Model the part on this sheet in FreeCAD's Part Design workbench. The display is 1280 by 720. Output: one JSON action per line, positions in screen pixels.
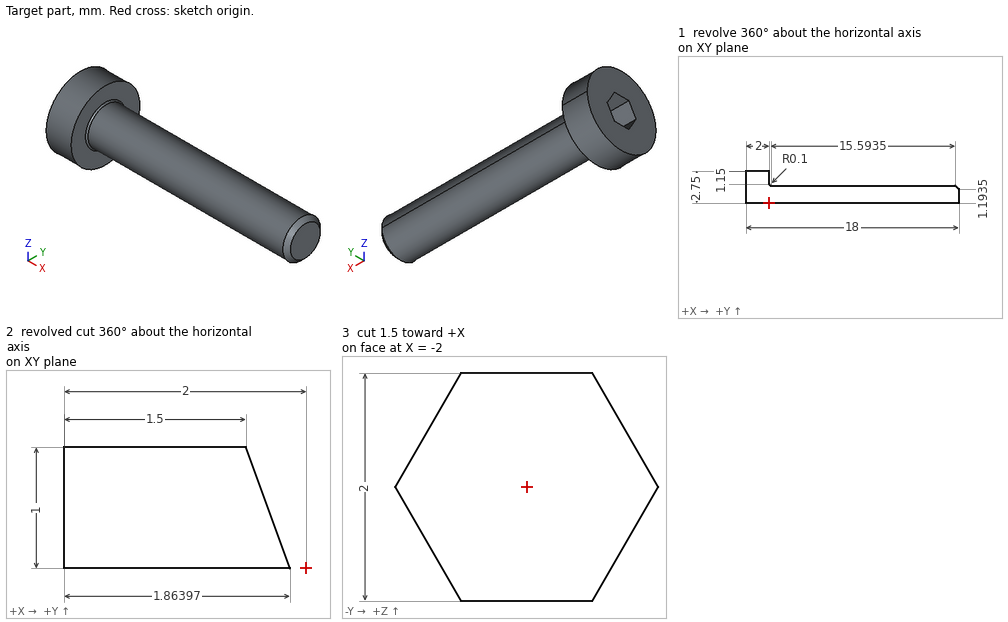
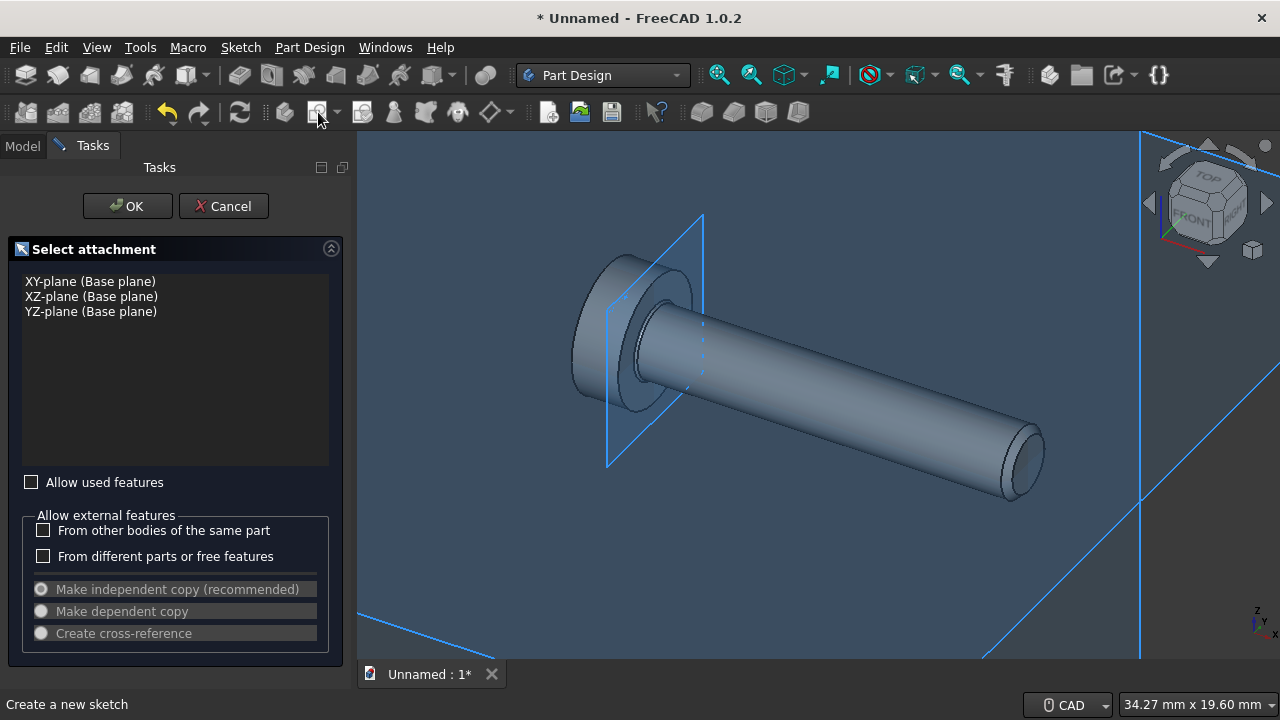
{"action": "left_click", "coordinate": [82, 282]}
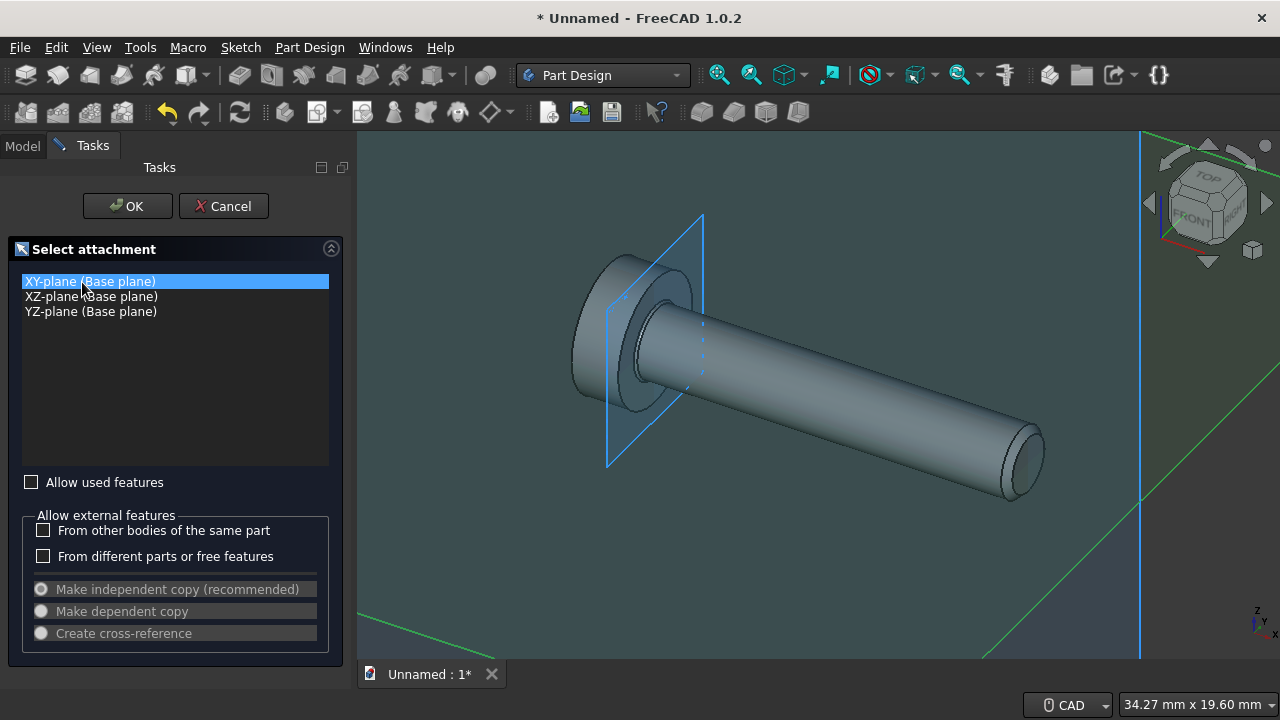
{"action": "left_click", "coordinate": [128, 206]}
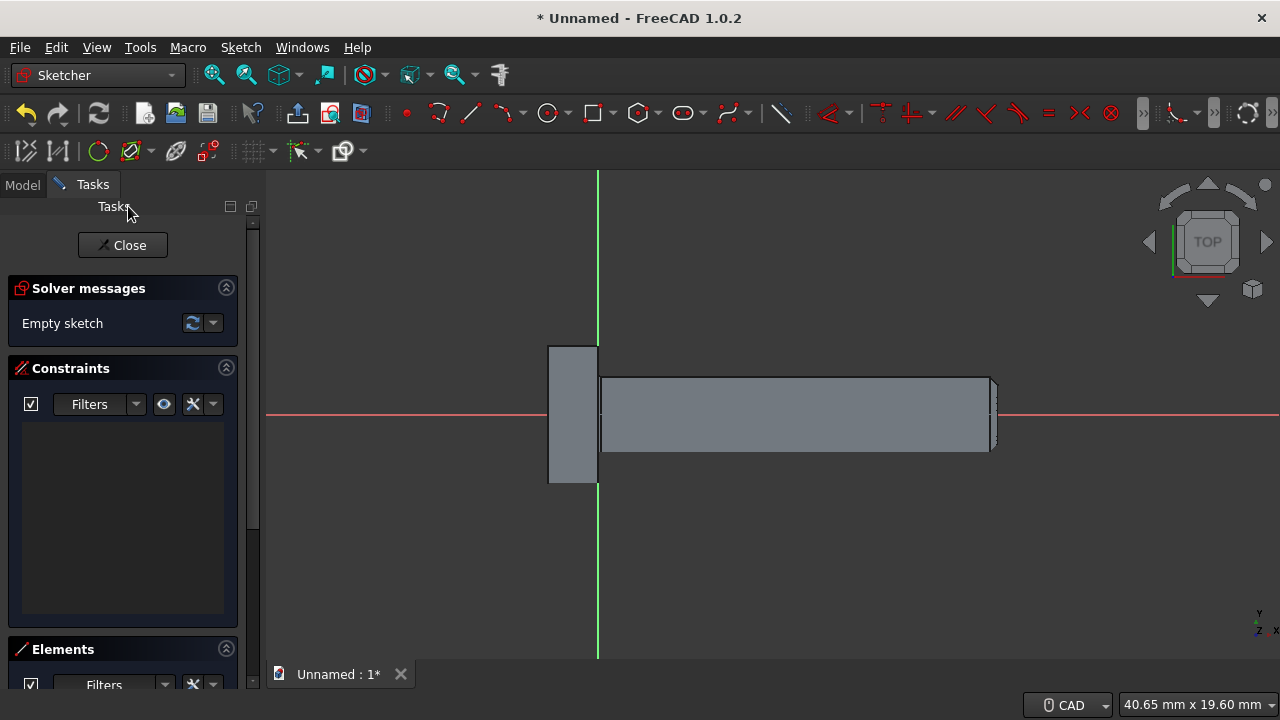
{"action": "left_click", "coordinate": [362, 114]}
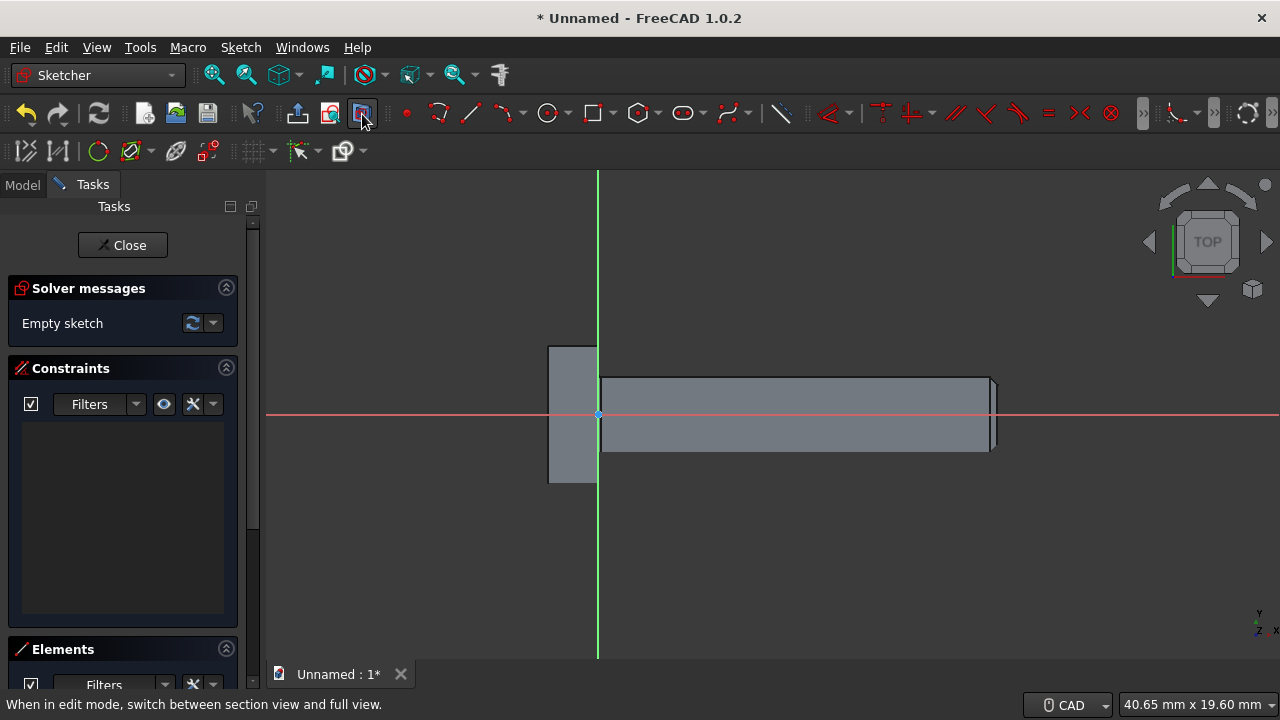
{"action": "scroll", "coordinate": [560, 401], "scroll_direction": "up", "scroll_amount": 12}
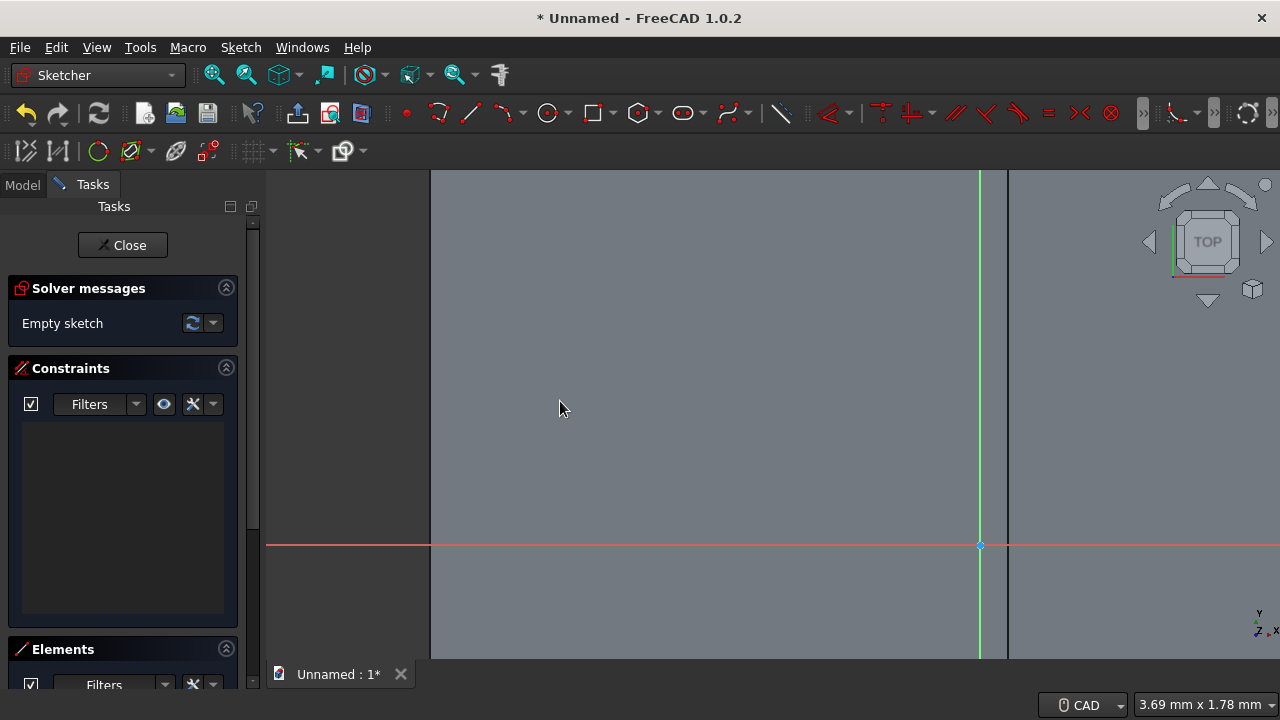
{"action": "left_click", "coordinate": [440, 114]}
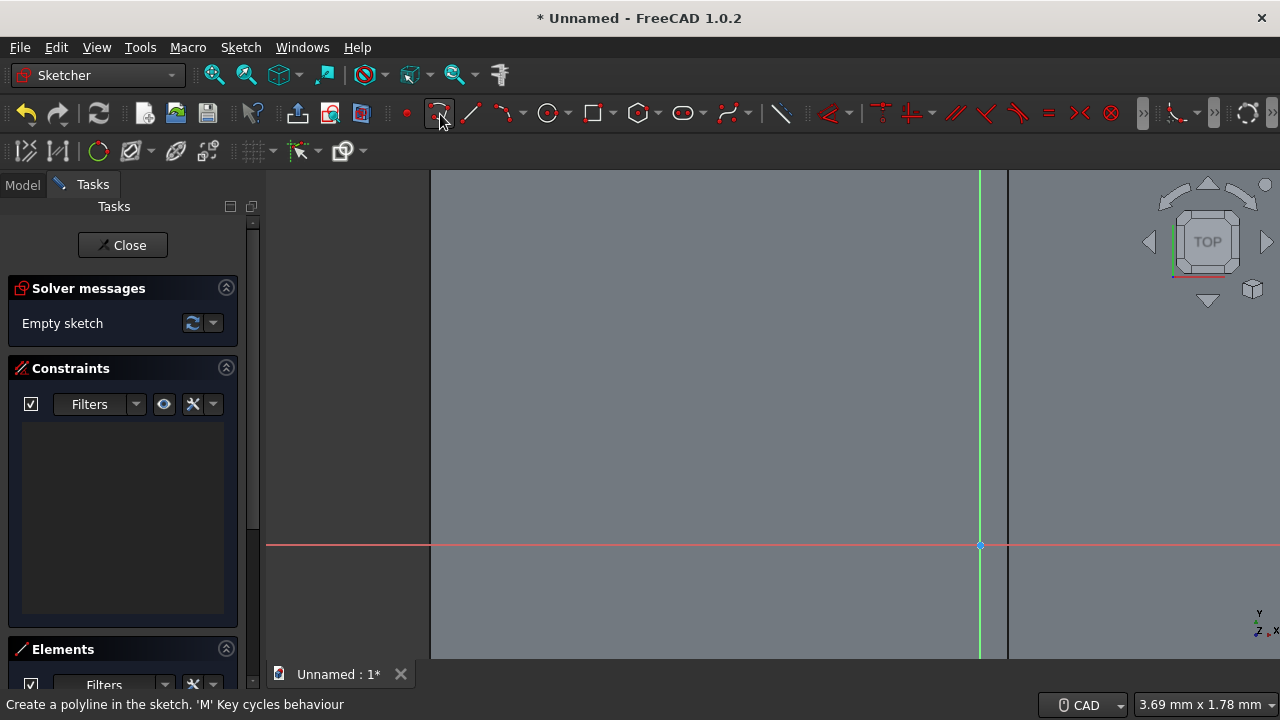
{"action": "left_click", "coordinate": [943, 545]}
{"action": "left_click", "coordinate": [843, 270]}
{"action": "left_click", "coordinate": [430, 270]}
{"action": "left_click", "coordinate": [430, 536]}
{"action": "left_click", "coordinate": [943, 545]}
{"action": "key", "text": "Escape"}
{"action": "key", "text": "Escape"}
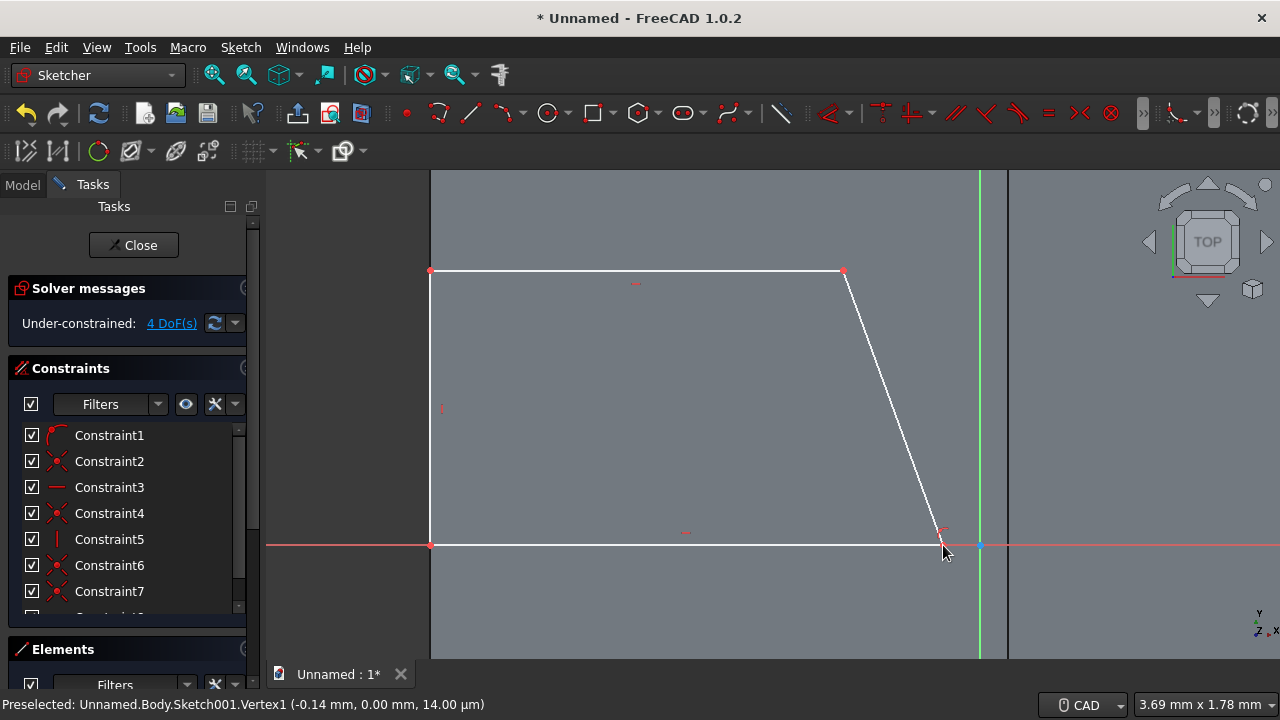
{"action": "left_click", "coordinate": [828, 114]}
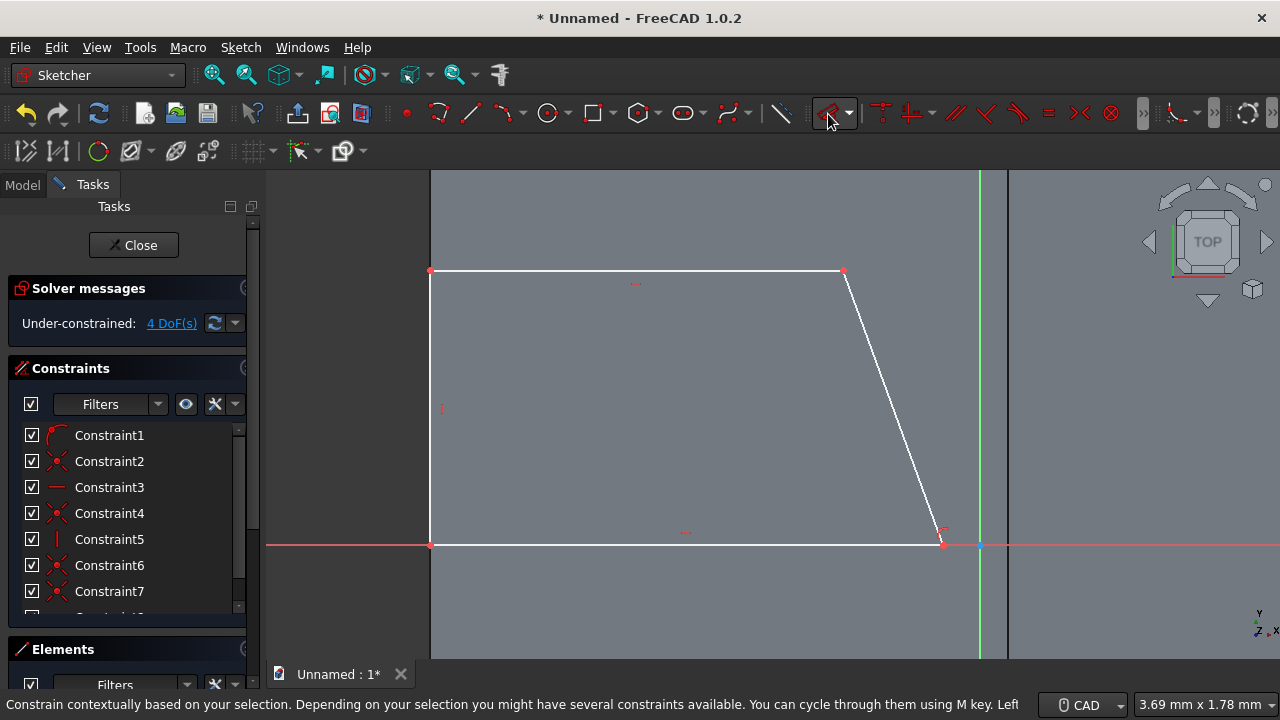
{"action": "left_click", "coordinate": [430, 353]}
{"action": "left_click", "coordinate": [396, 408]}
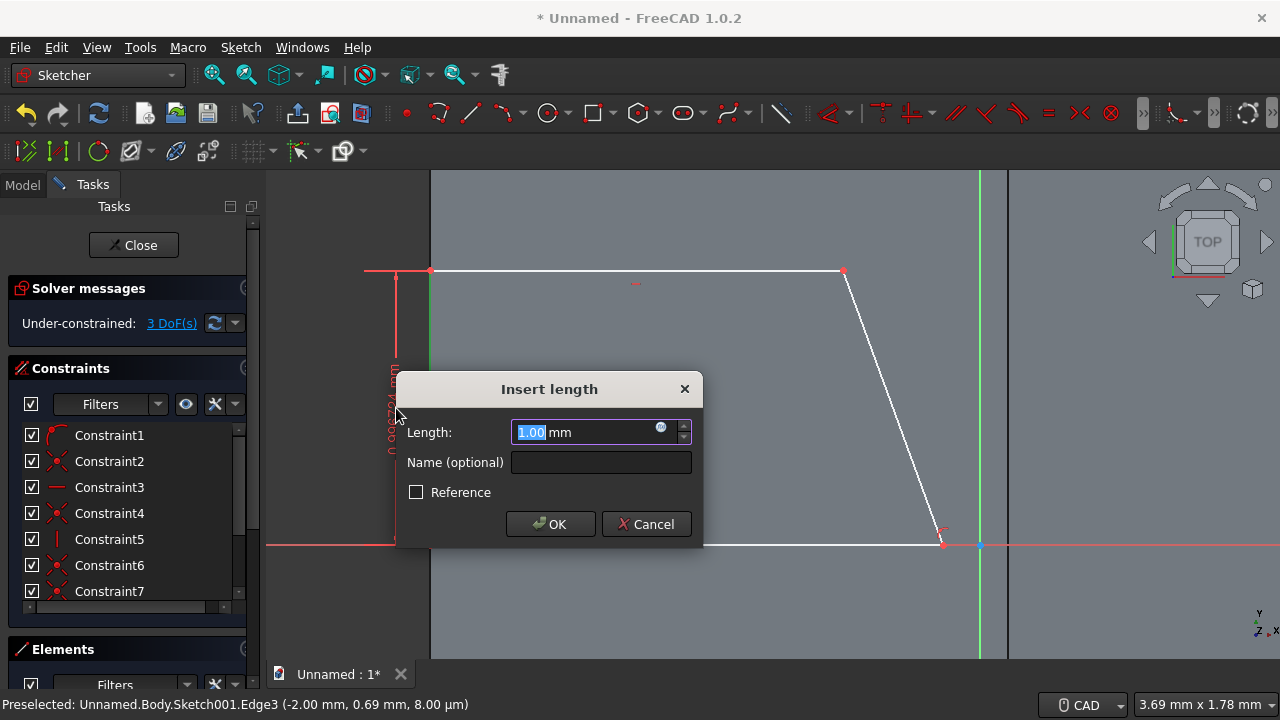
{"action": "type", "text": "1"}
{"action": "key", "text": "Return"}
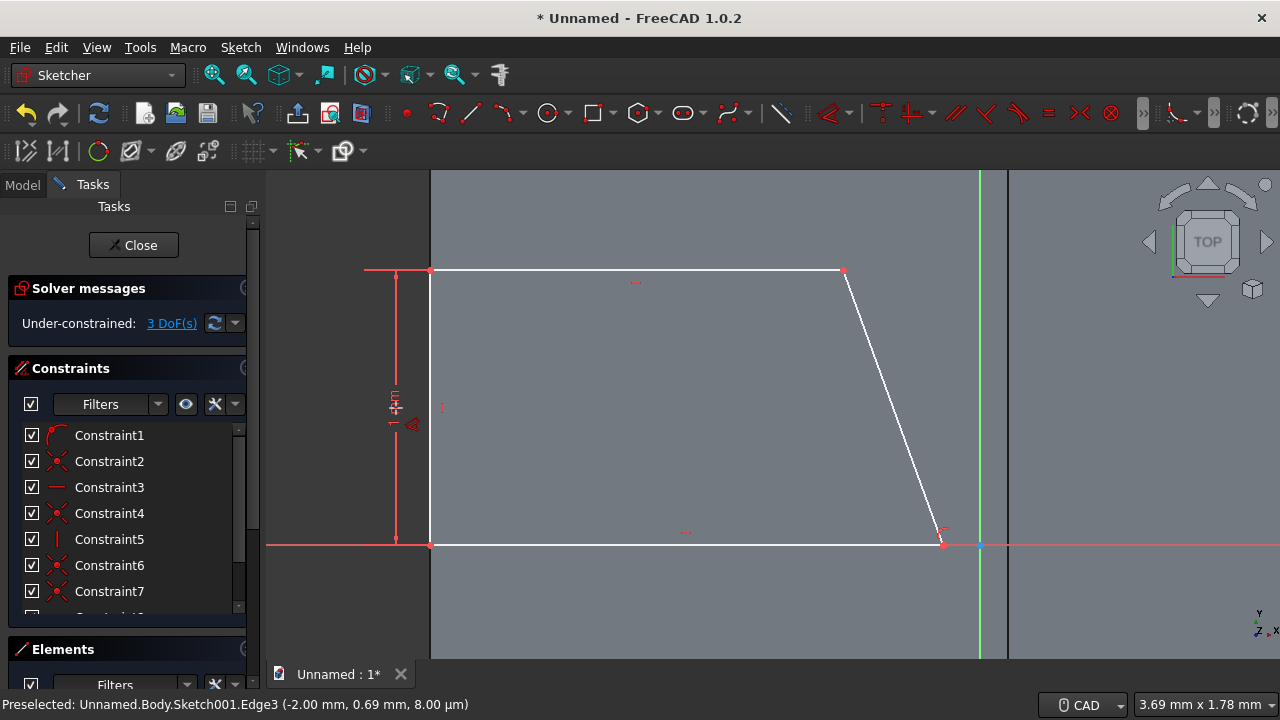
{"action": "left_click", "coordinate": [430, 270]}
{"action": "left_click", "coordinate": [705, 579]}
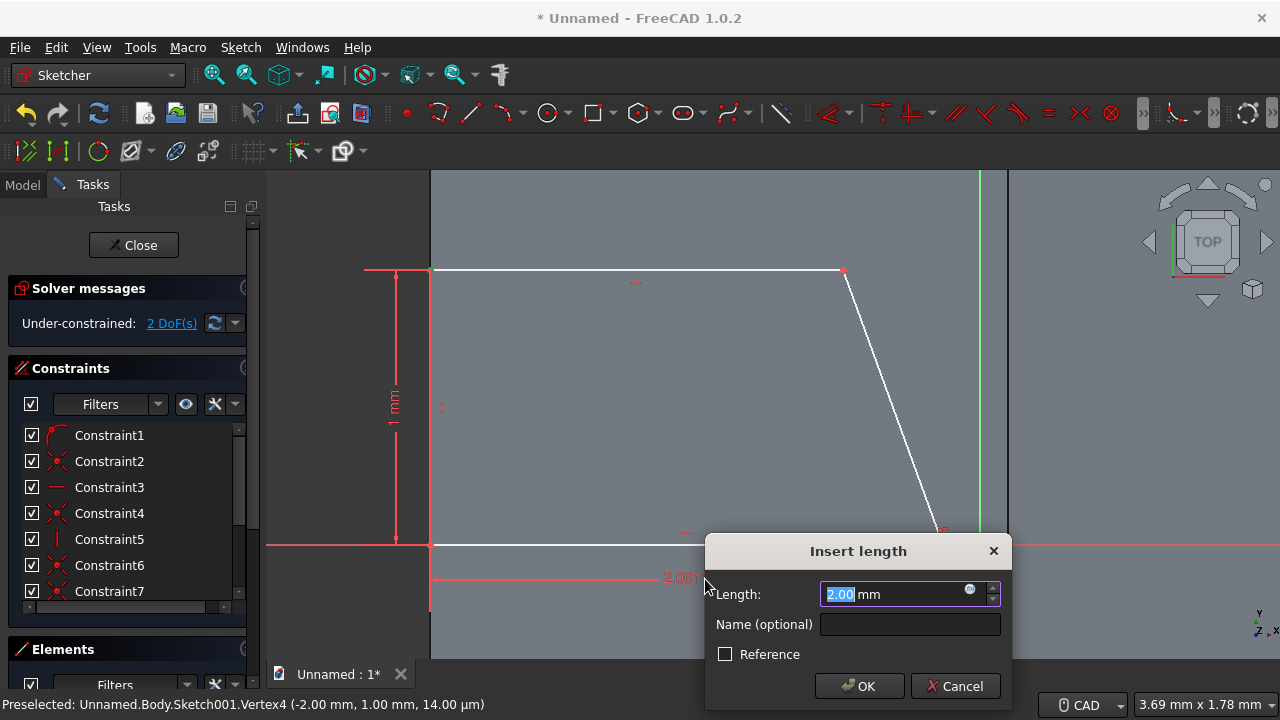
{"action": "type", "text": "2"}
{"action": "key", "text": "Return"}